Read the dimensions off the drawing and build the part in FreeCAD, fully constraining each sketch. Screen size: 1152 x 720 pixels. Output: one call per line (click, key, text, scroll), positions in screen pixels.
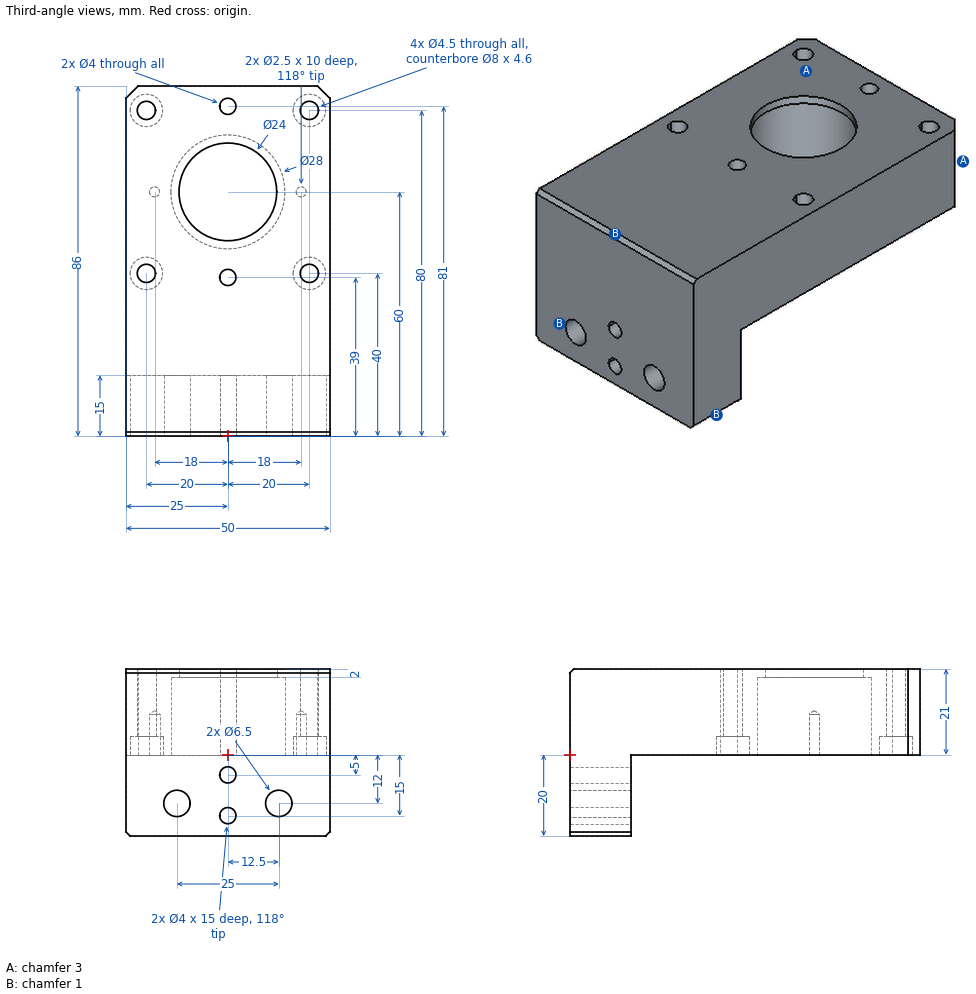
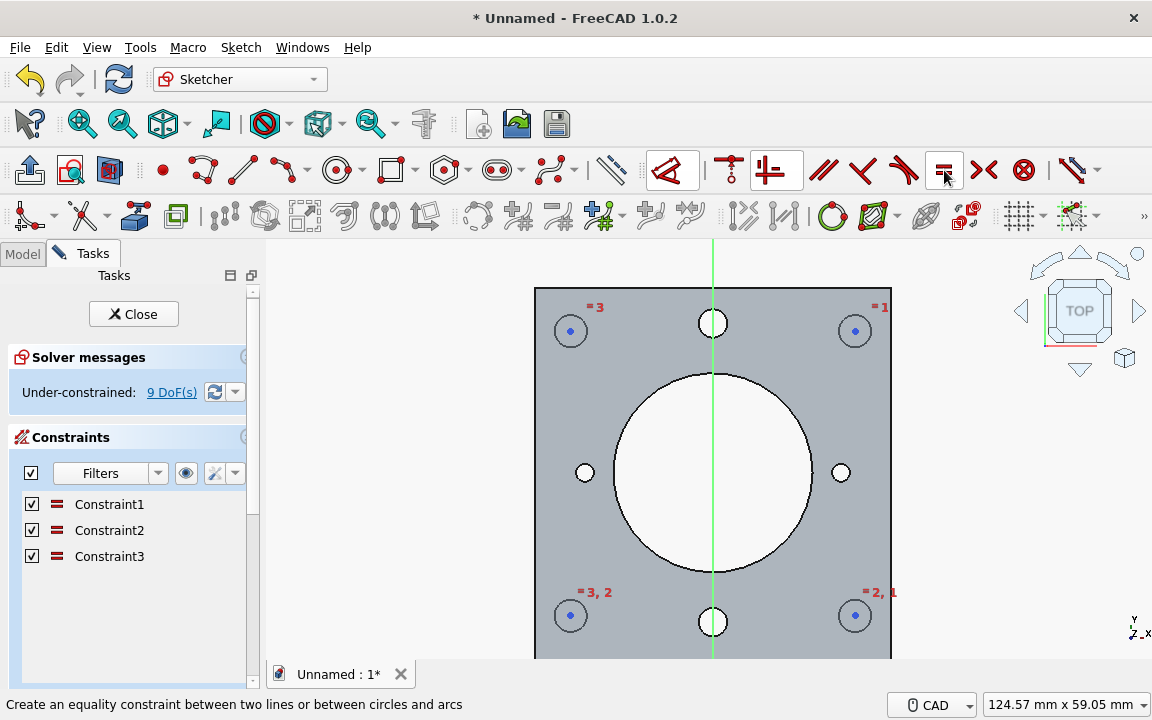
click(855, 331)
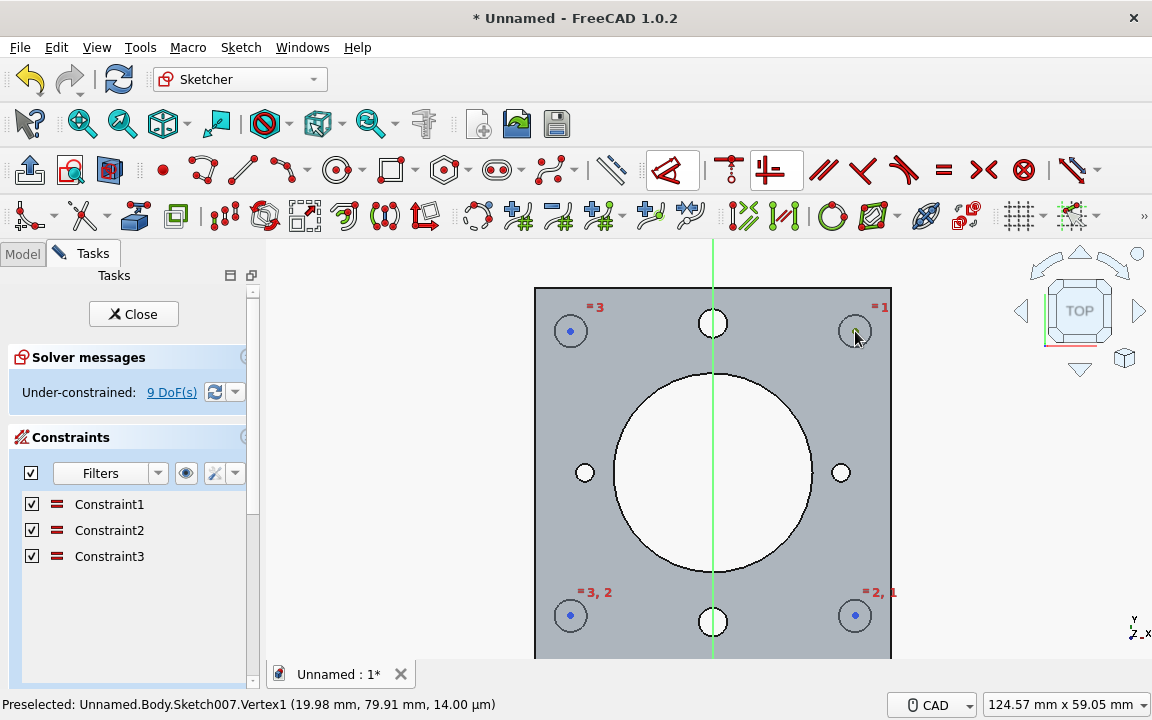
click(855, 616)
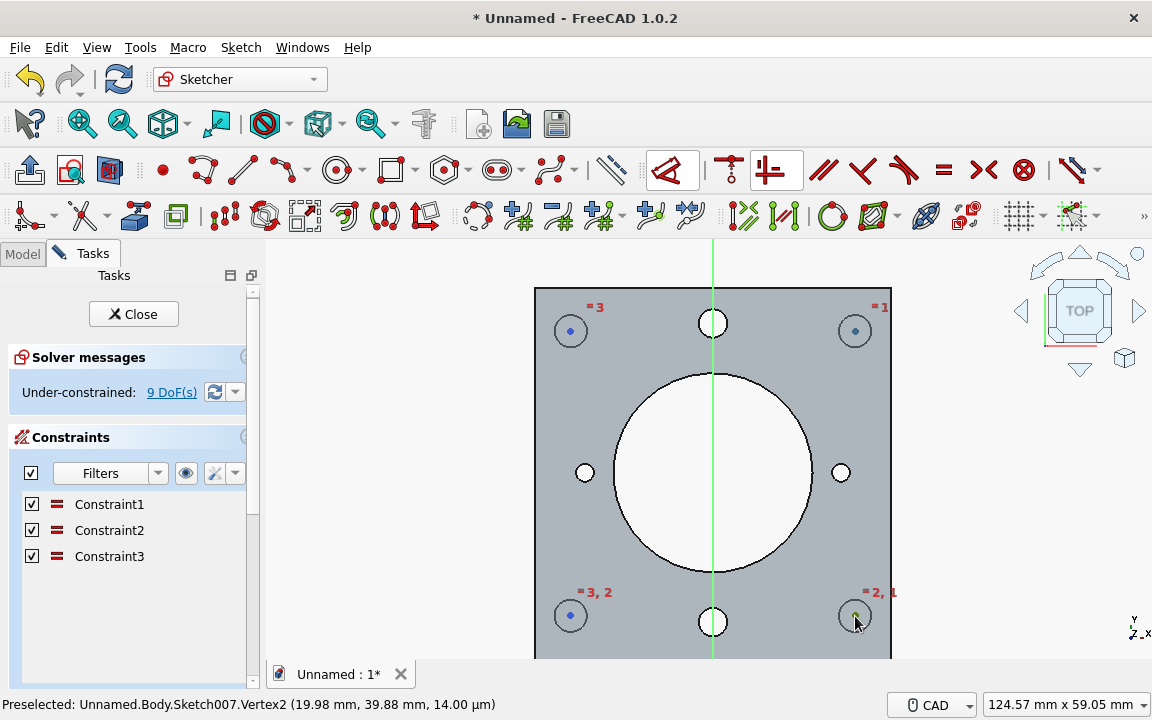
click(798, 170)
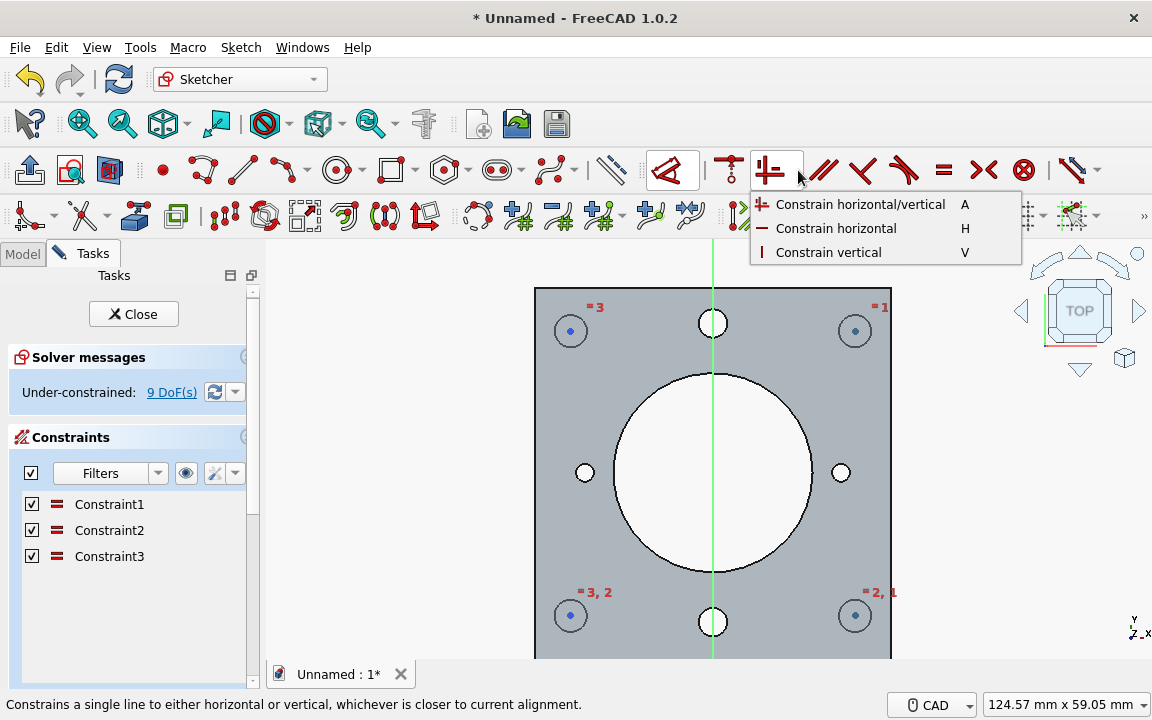
click(886, 252)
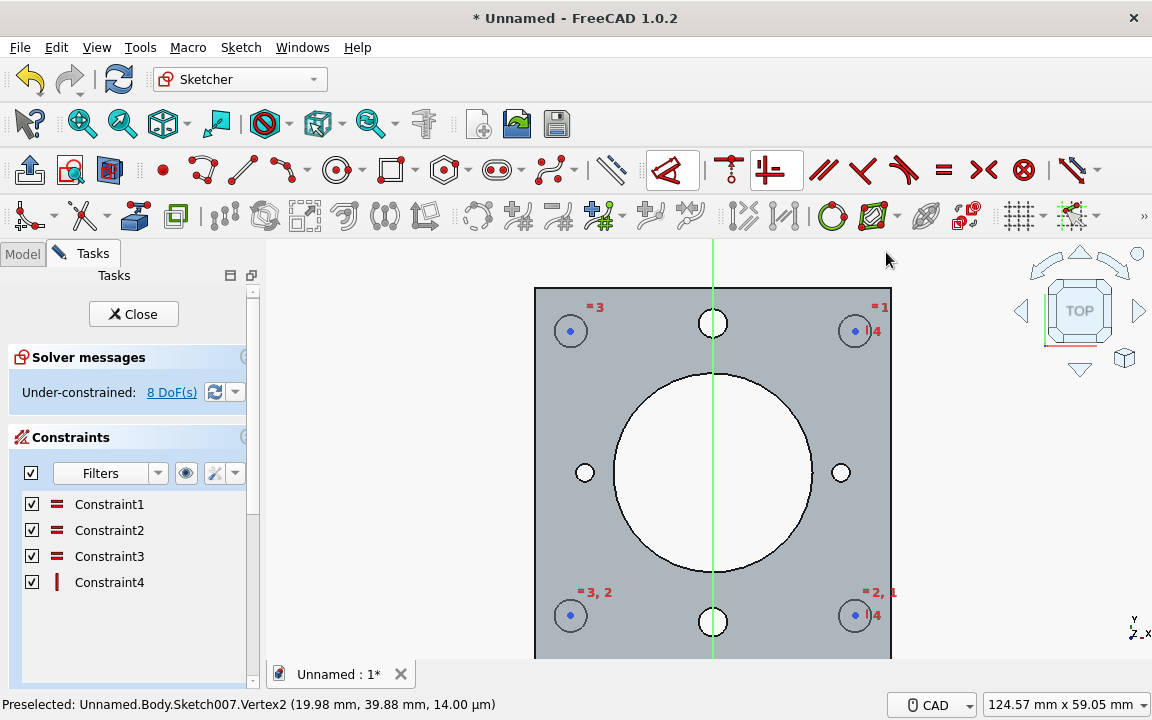
click(855, 616)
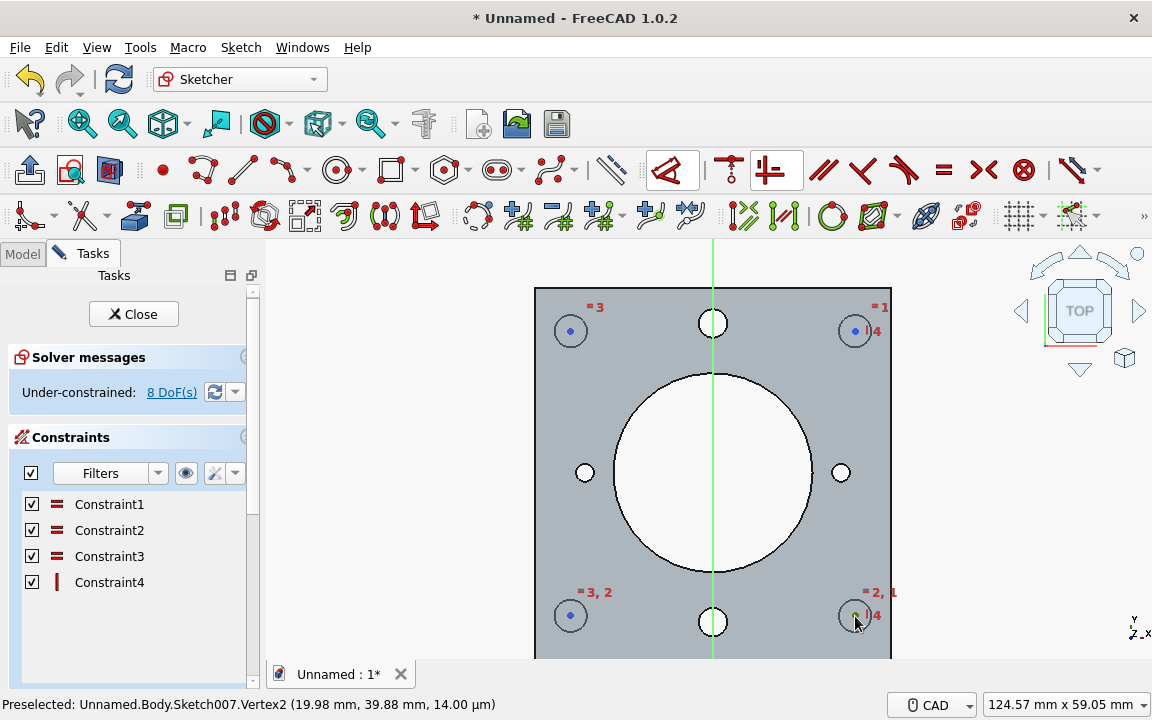
click(571, 616)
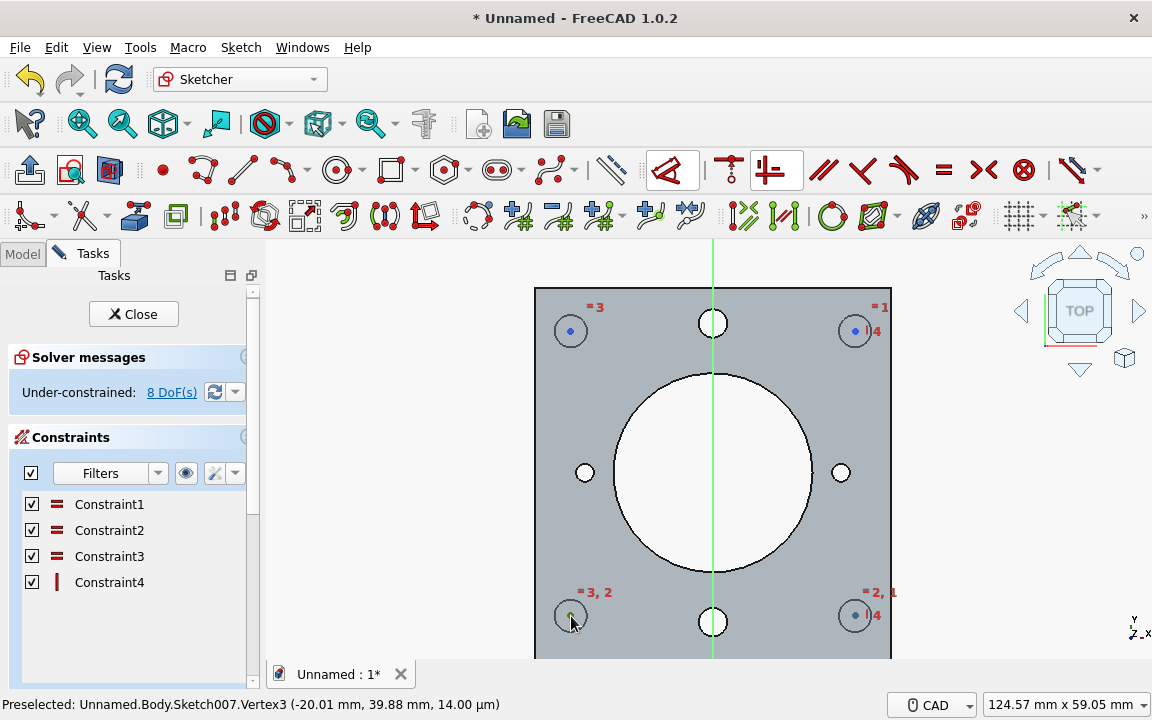
click(798, 170)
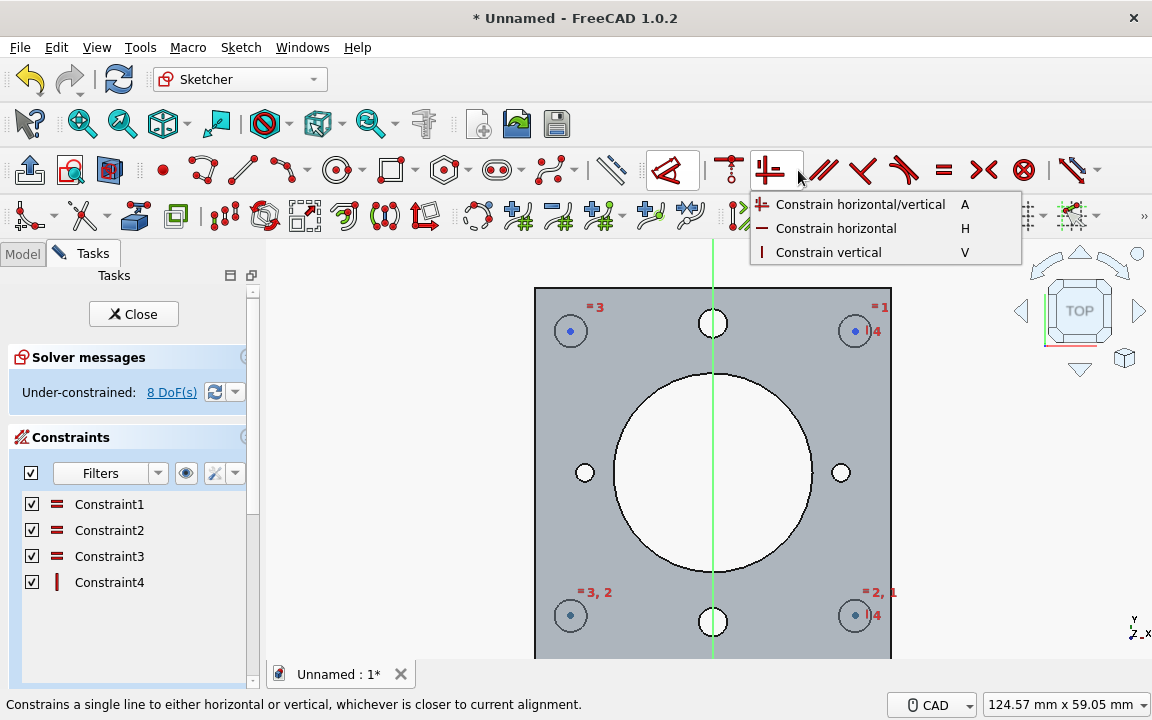
click(886, 228)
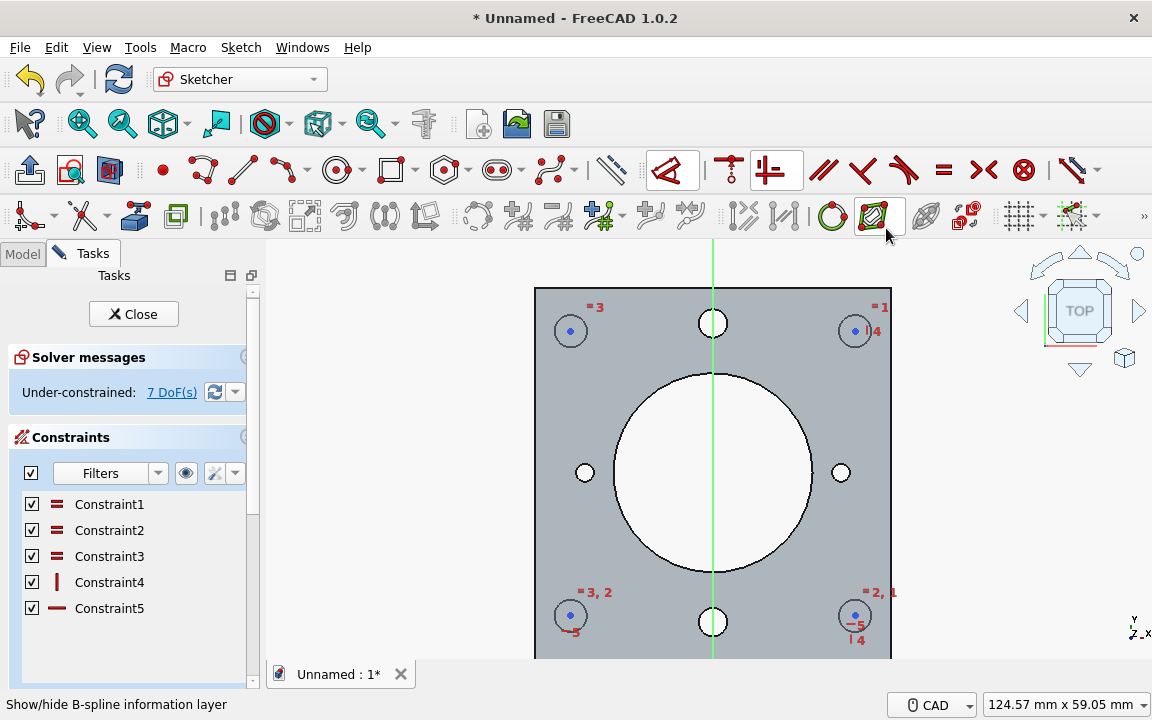
click(571, 616)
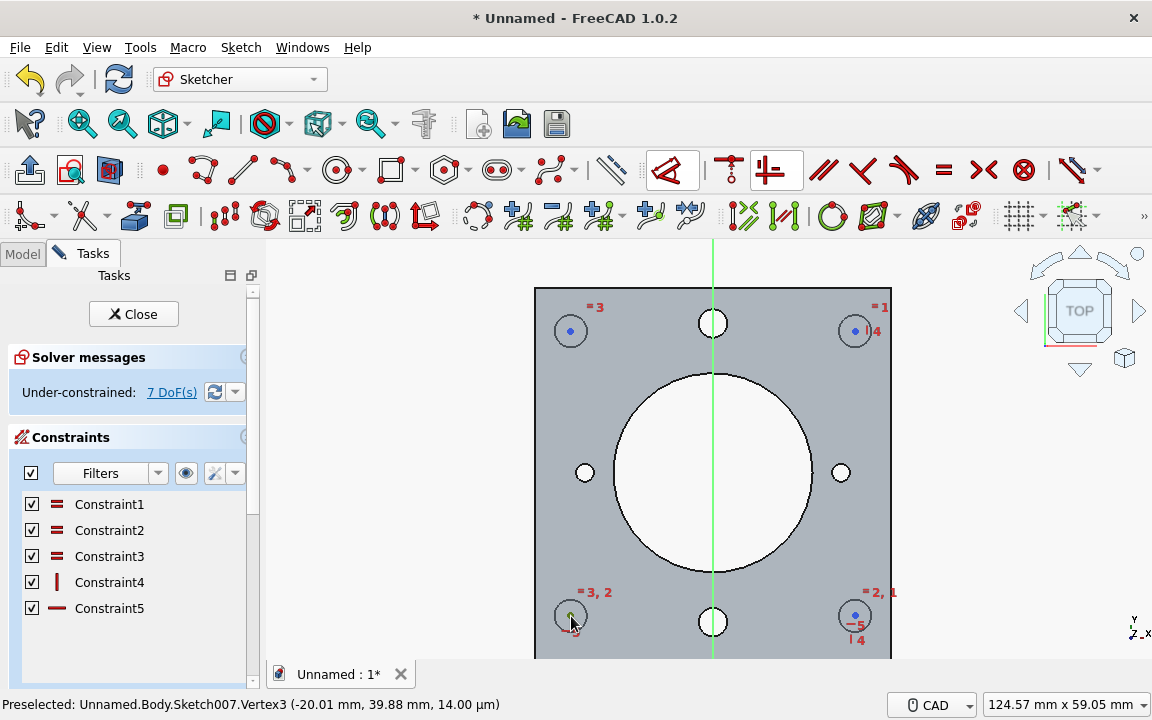
click(571, 331)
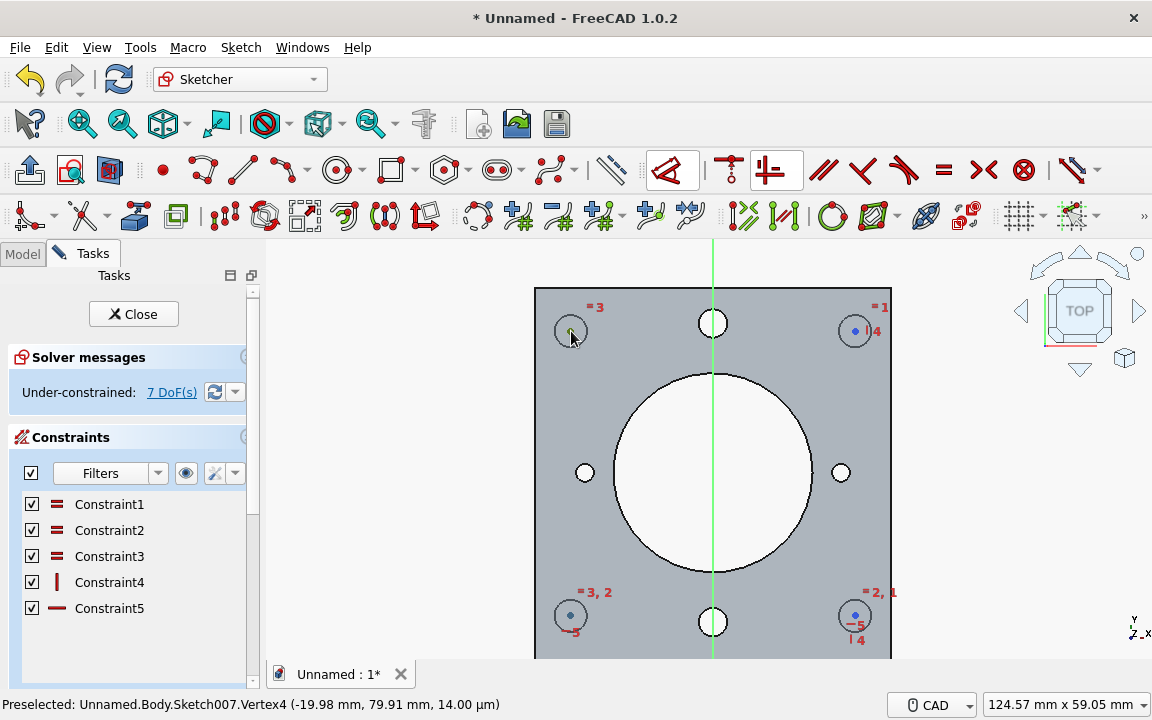
key(v)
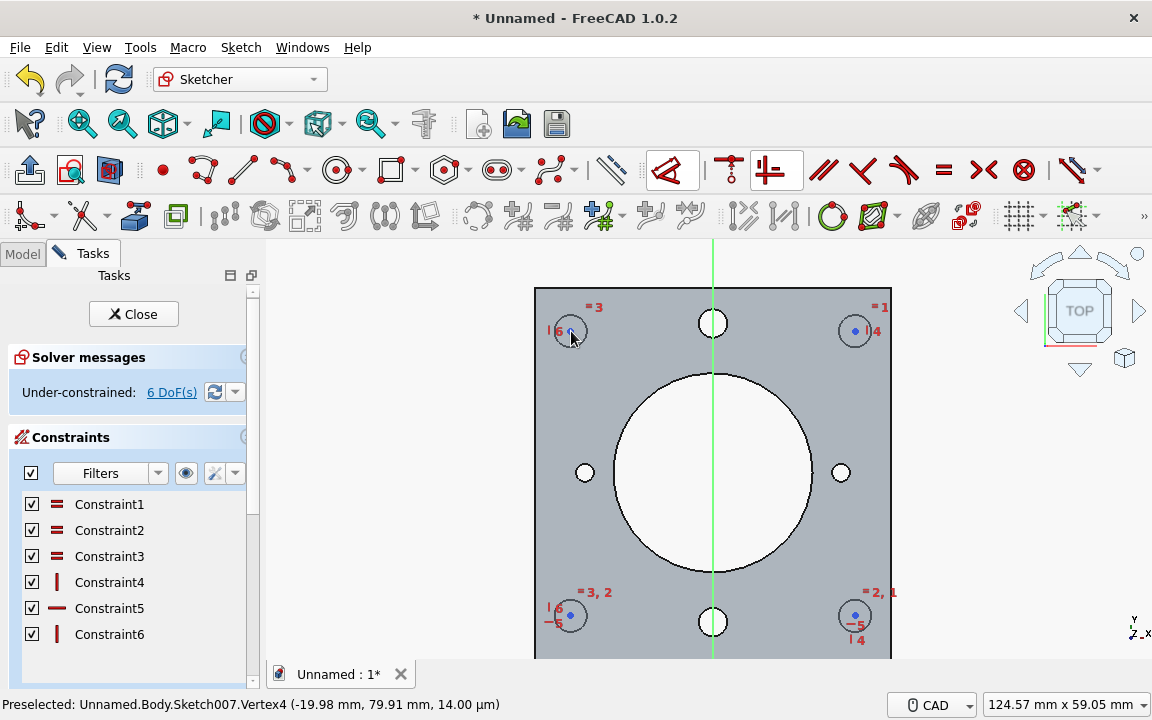
click(855, 331)